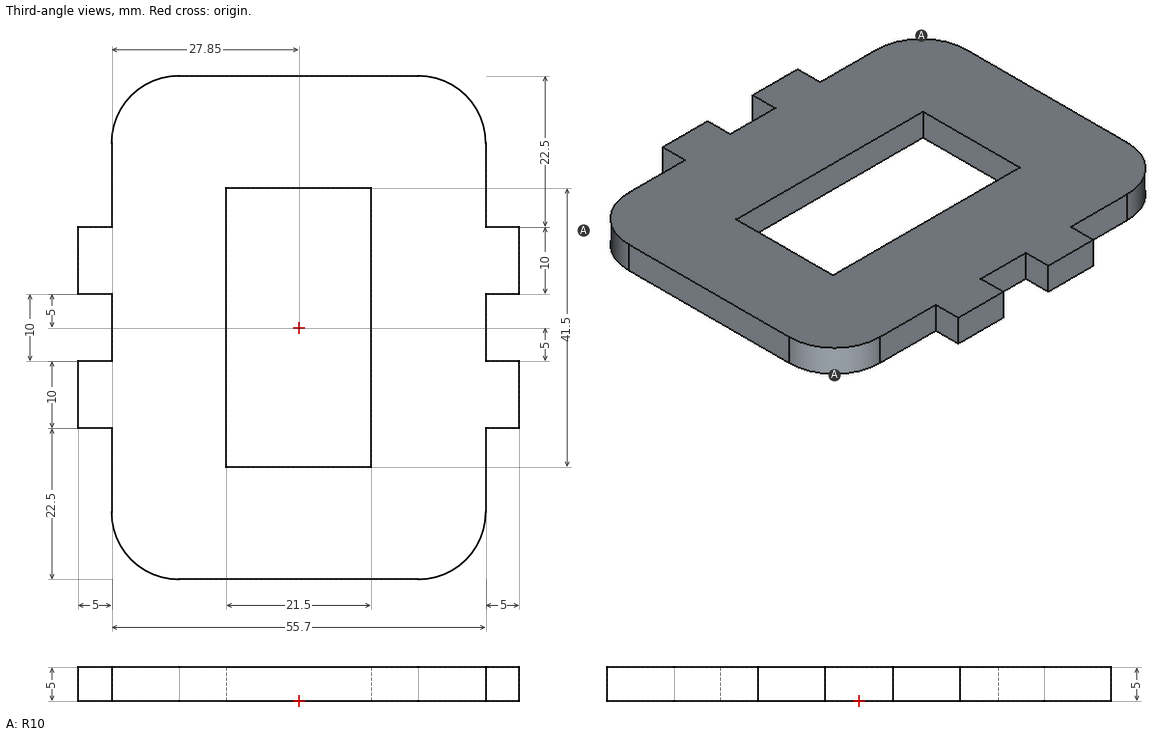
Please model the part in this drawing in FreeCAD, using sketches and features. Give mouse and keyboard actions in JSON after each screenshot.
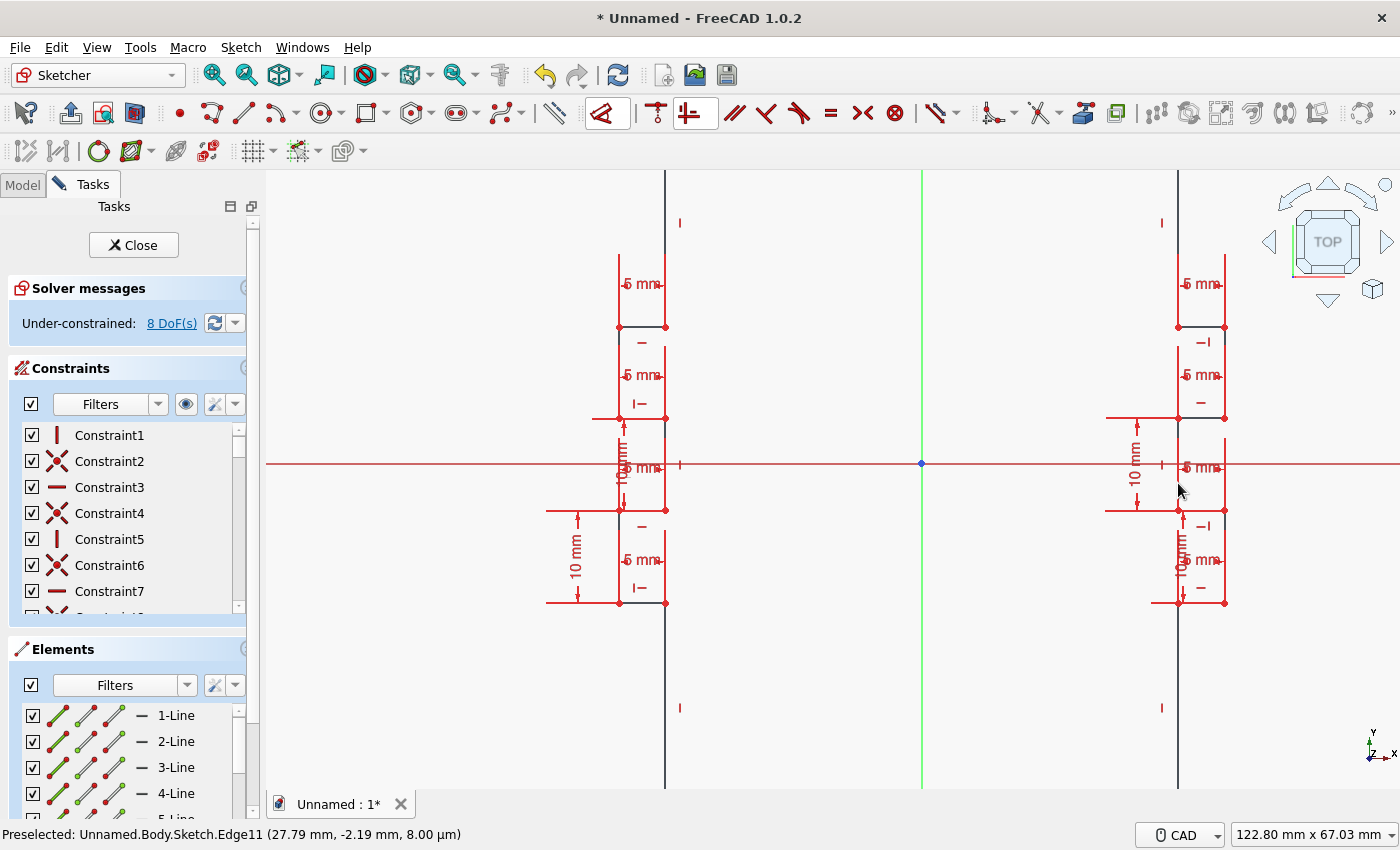
{"action": "left_click", "coordinate": [1225, 391]}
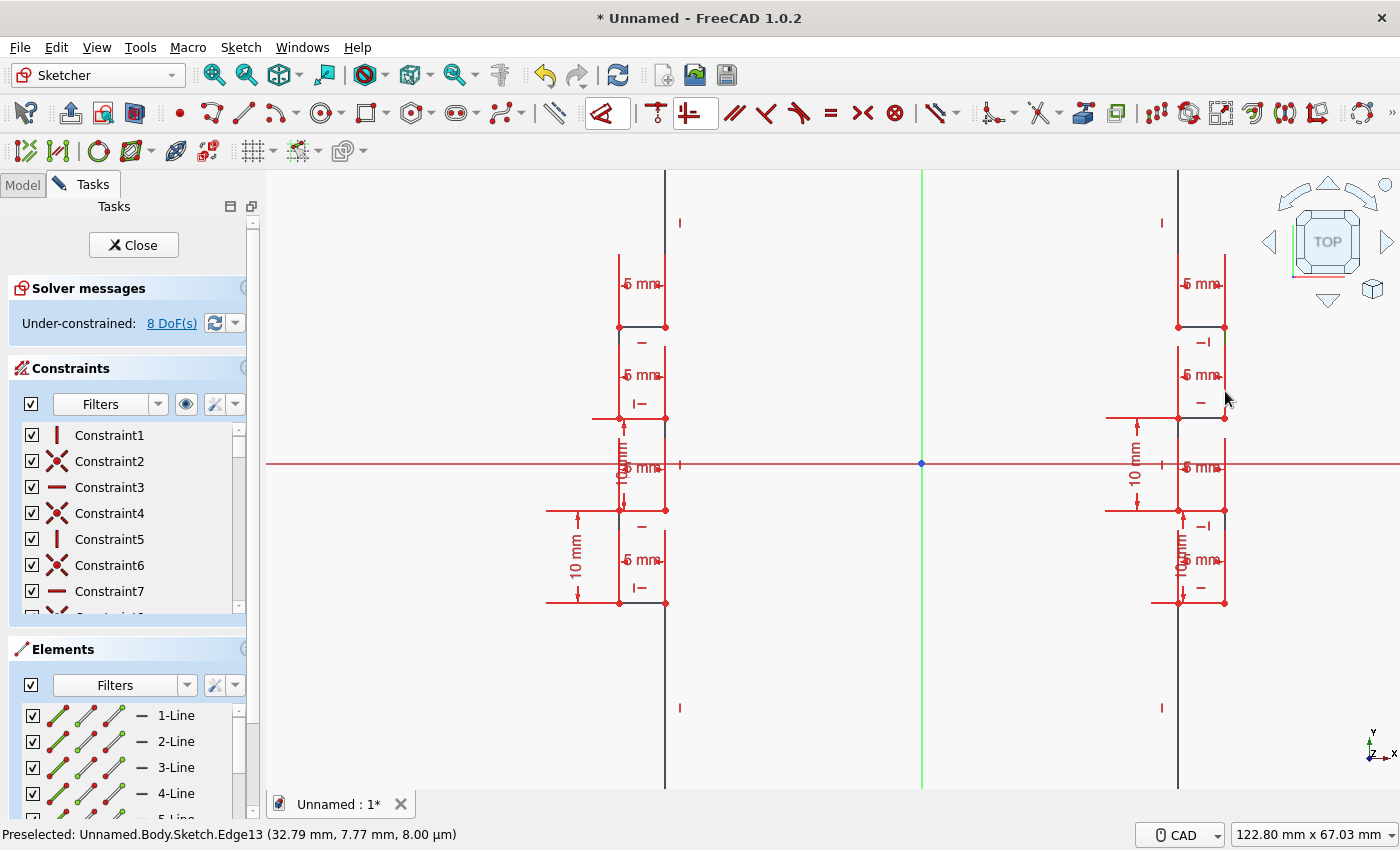
{"action": "key", "text": "i"}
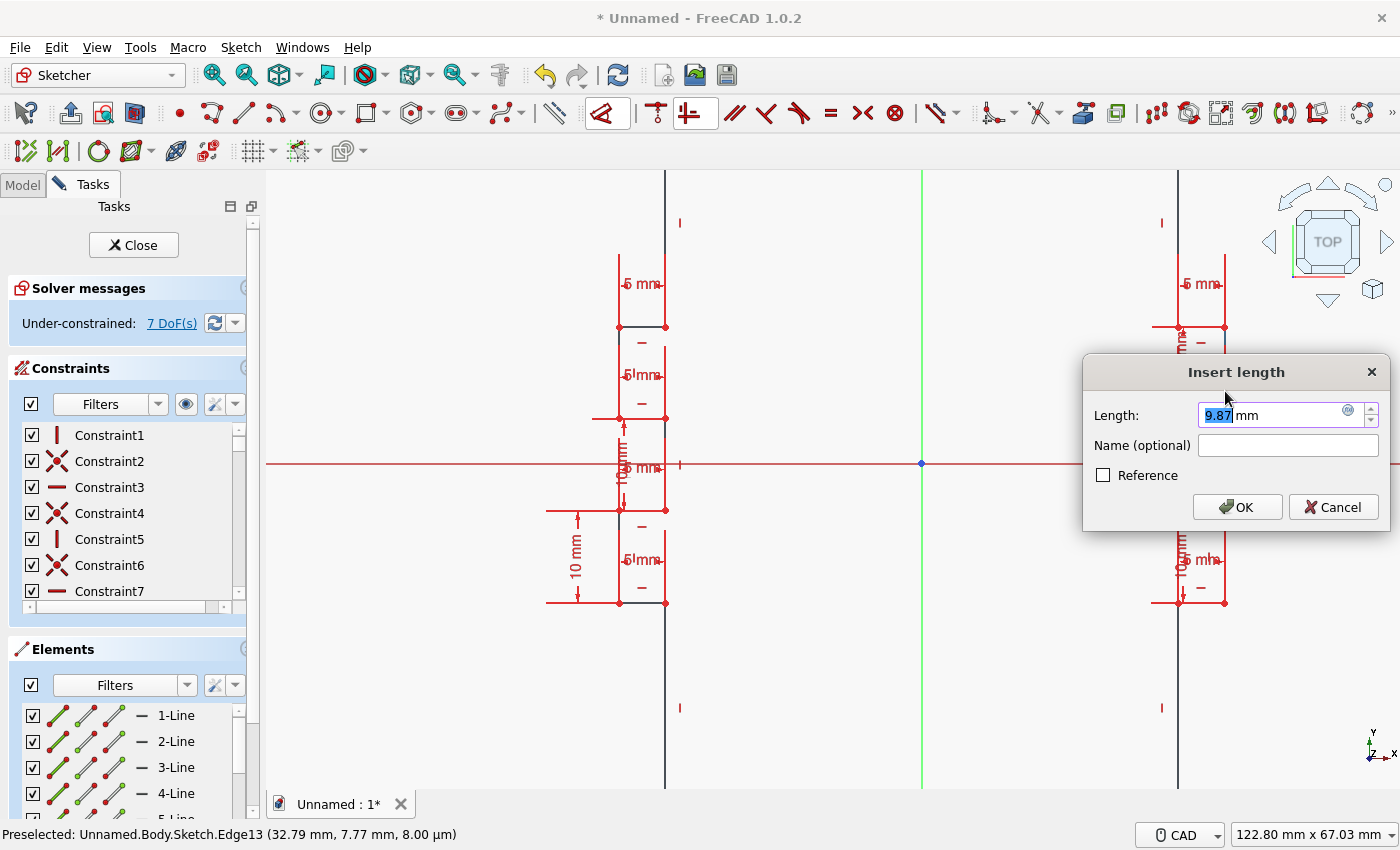
{"action": "type", "text": "10"}
{"action": "key", "text": "Return"}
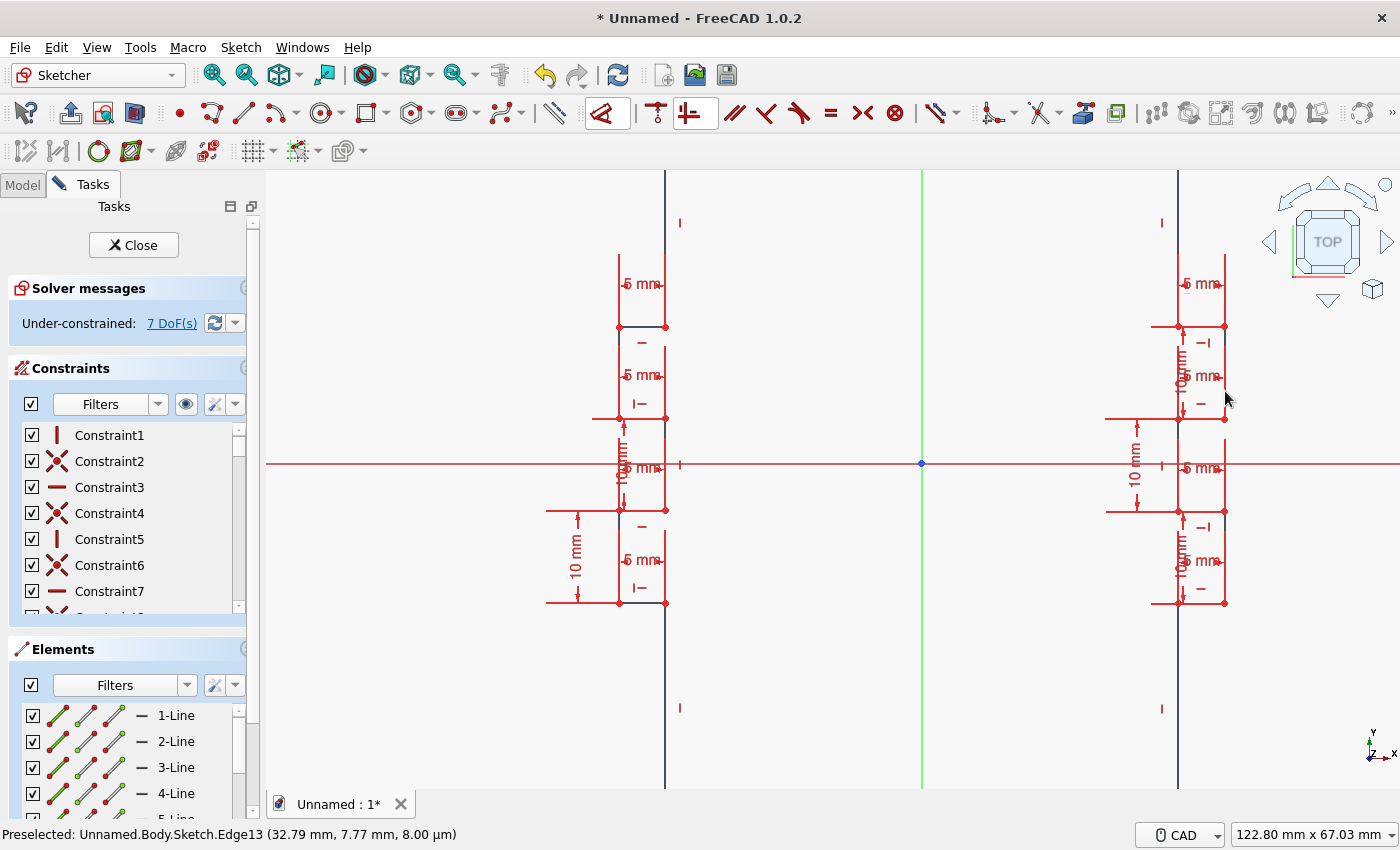
{"action": "left_click", "coordinate": [619, 355]}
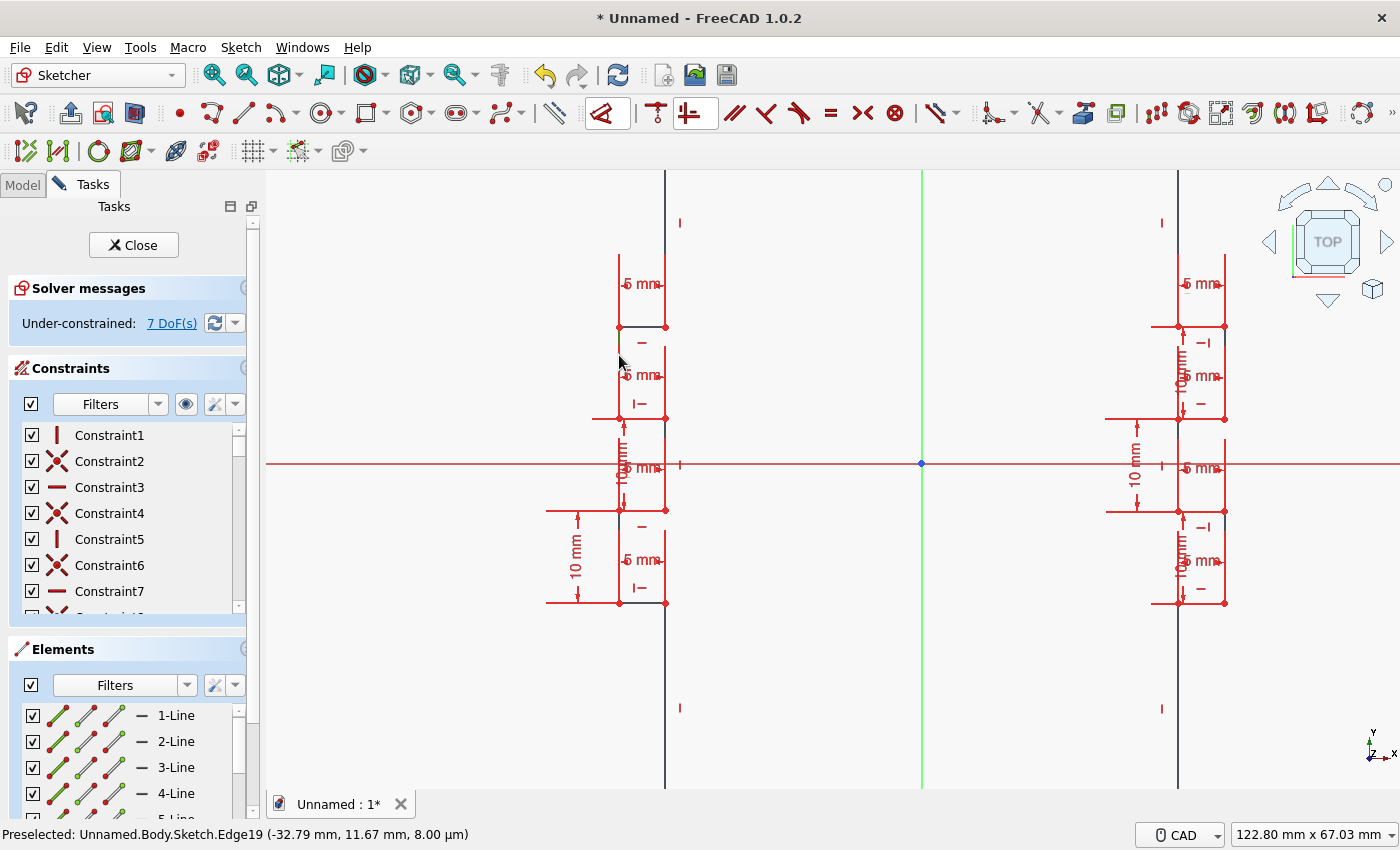
{"action": "key", "text": "i"}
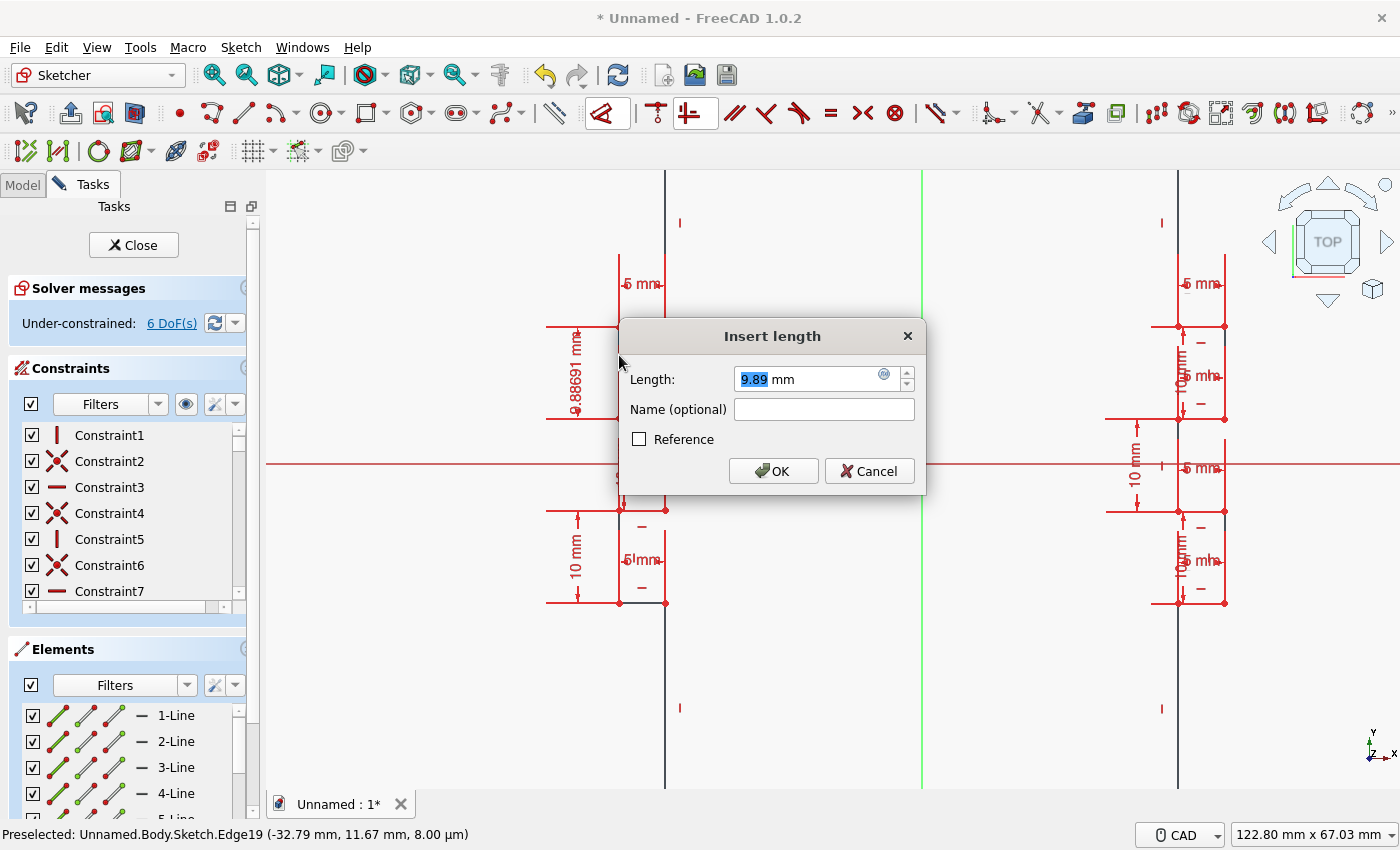
{"action": "type", "text": "10"}
{"action": "key", "text": "Return"}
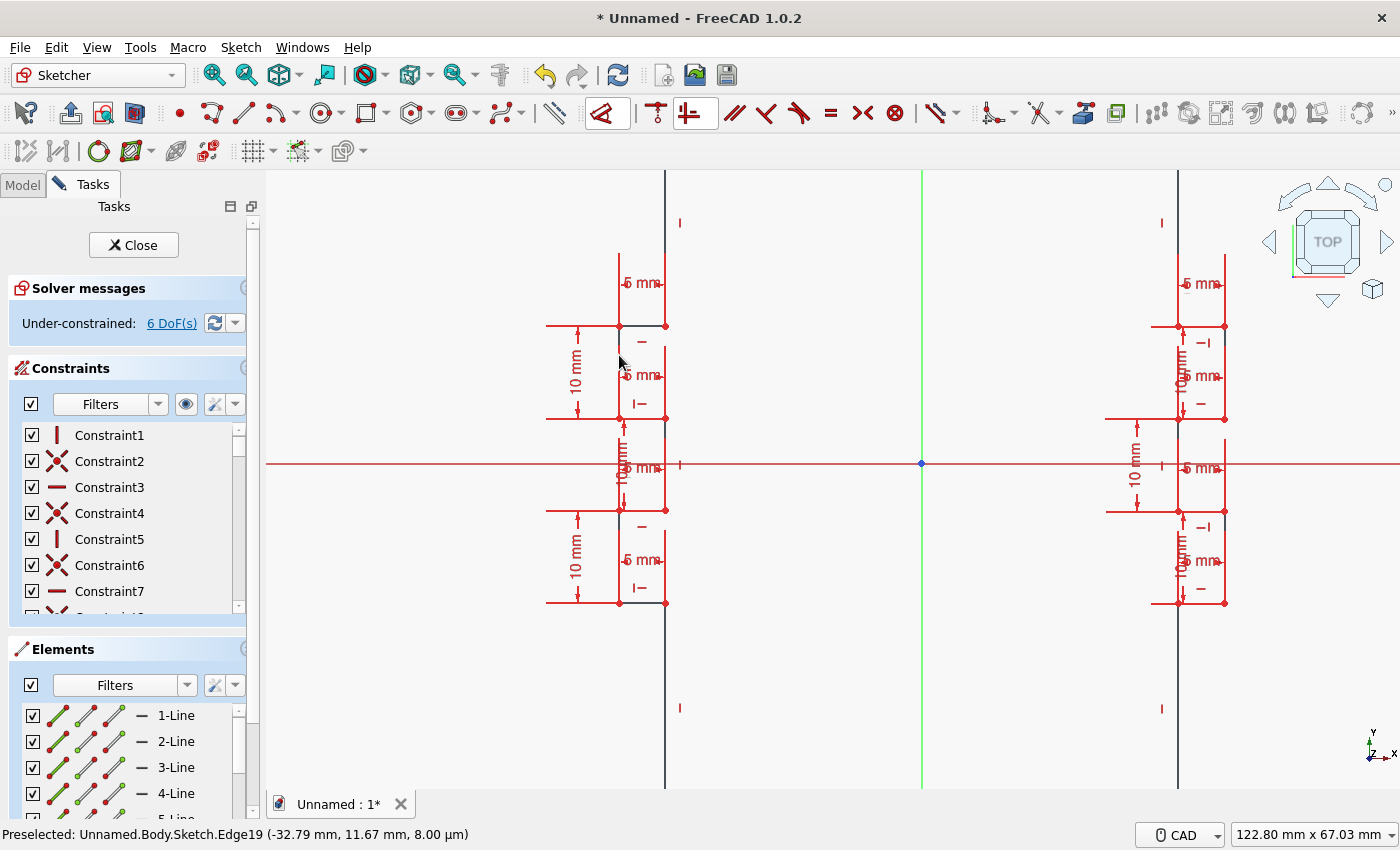
{"action": "left_click", "coordinate": [665, 419]}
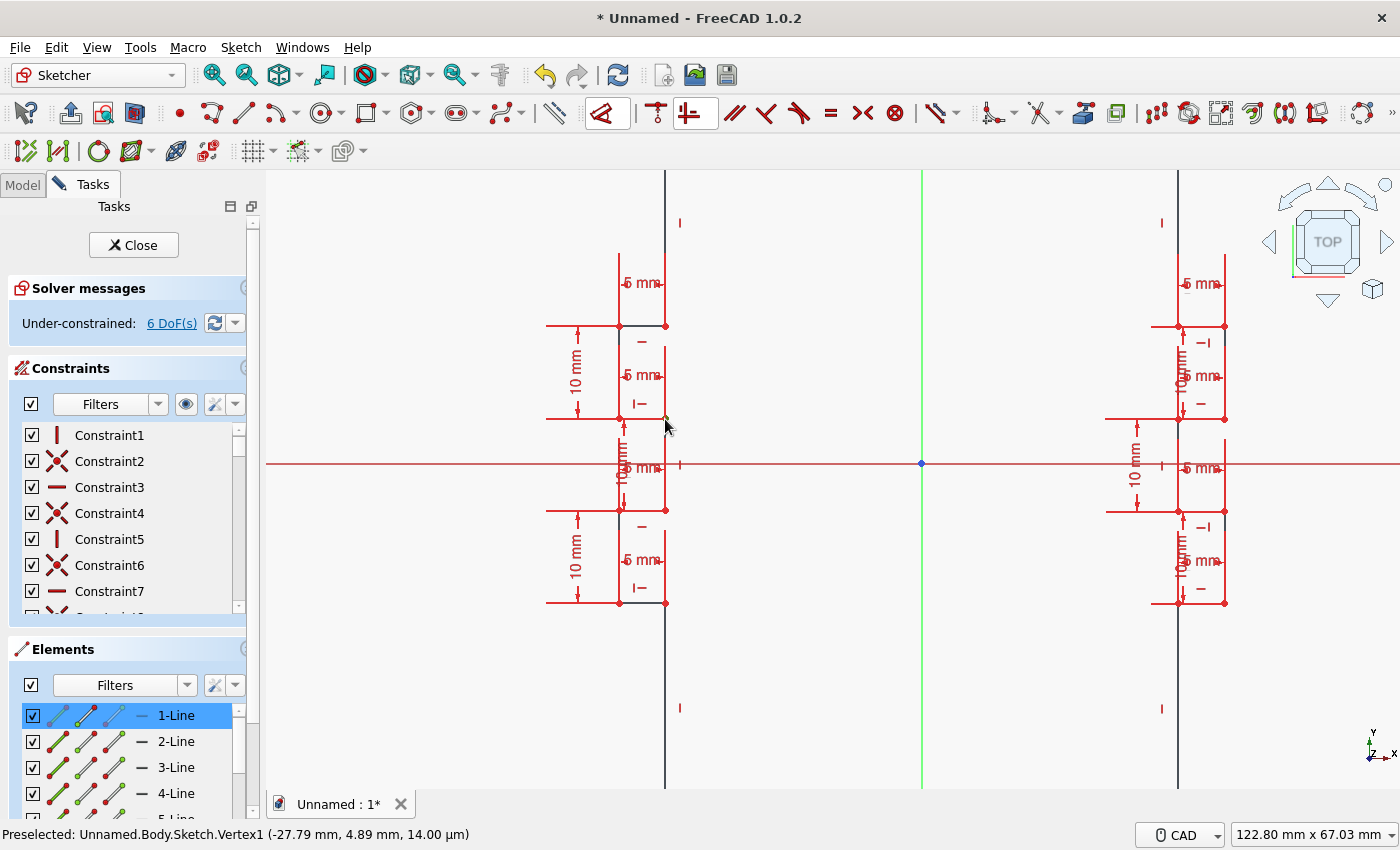
{"action": "key", "text": "i"}